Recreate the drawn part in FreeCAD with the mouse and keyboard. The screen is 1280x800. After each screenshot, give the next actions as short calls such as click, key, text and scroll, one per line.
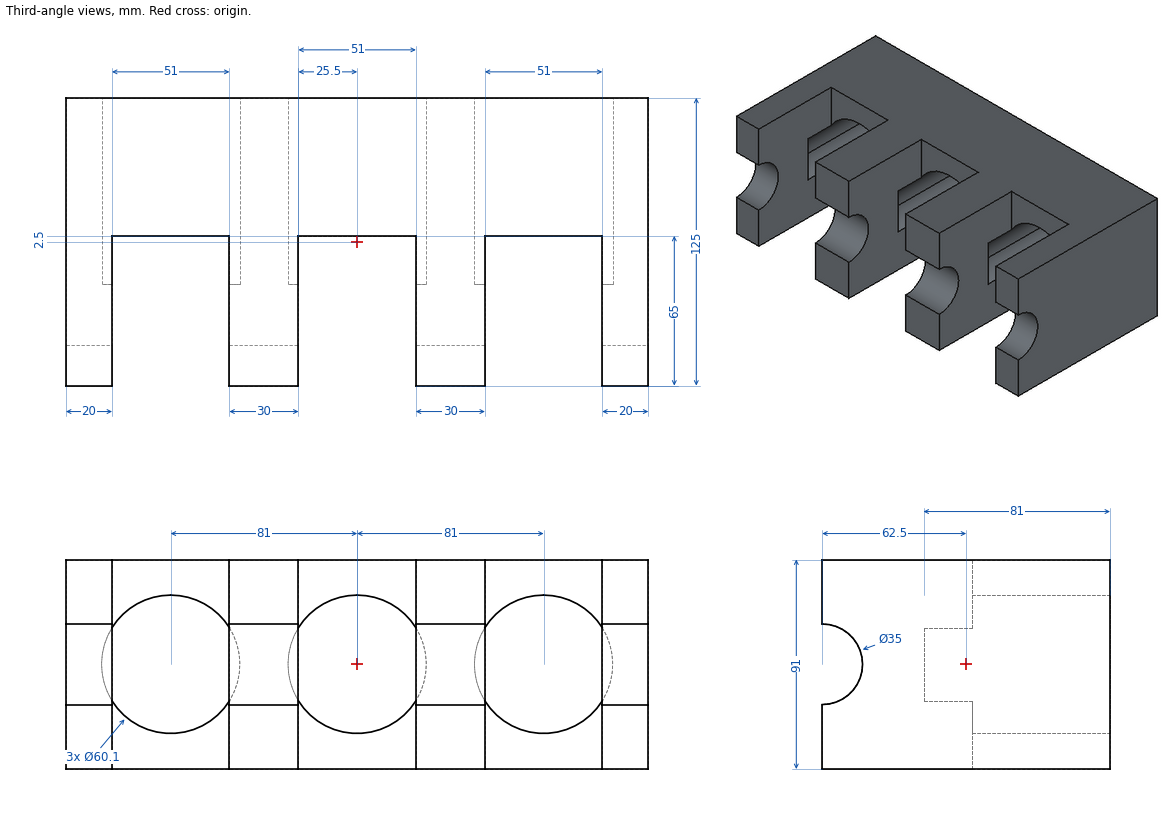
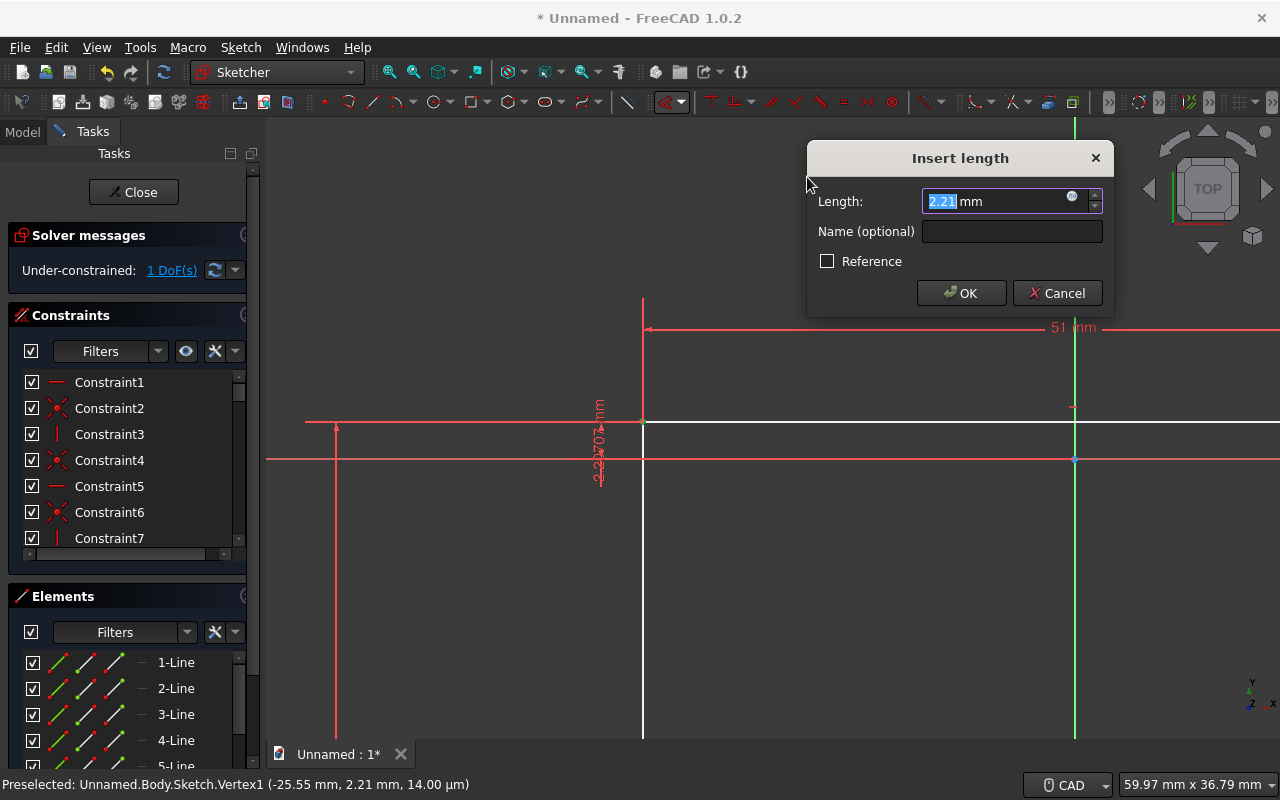
text(2.5)
key(Return)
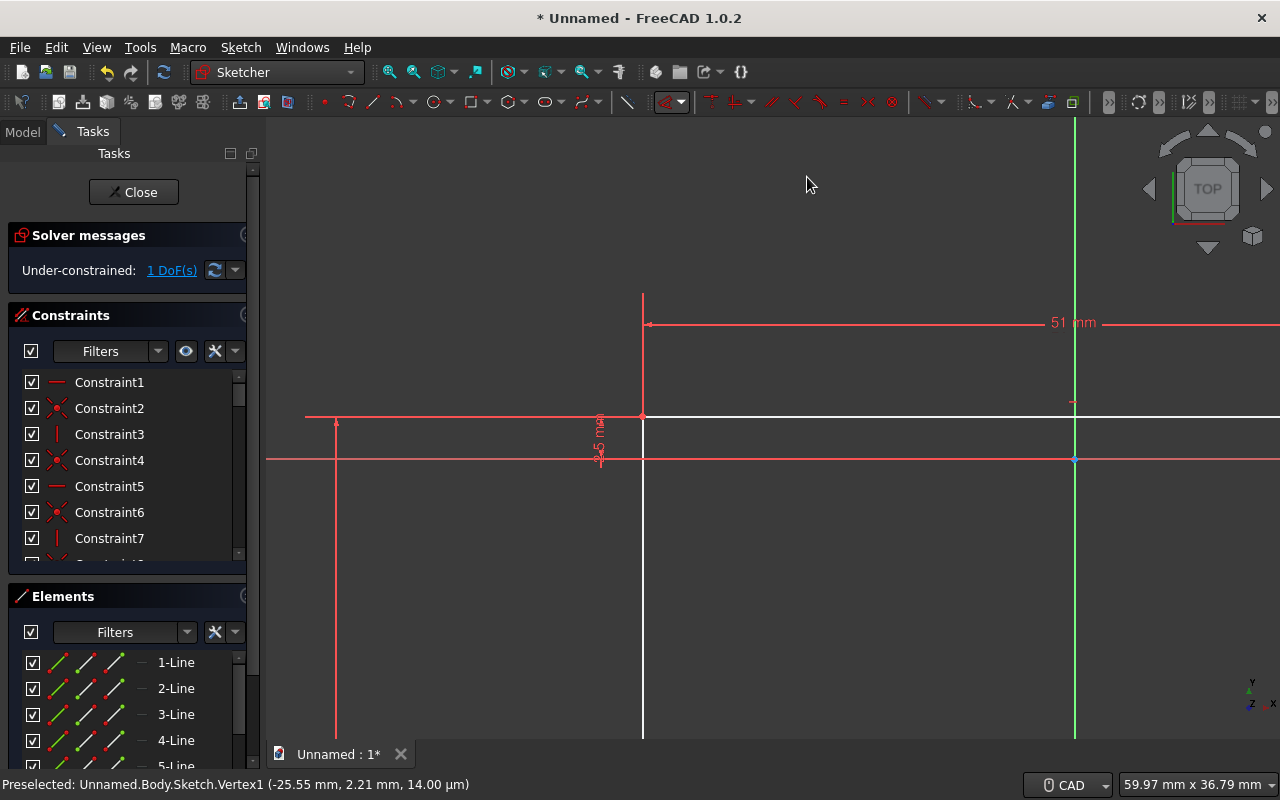
scroll(647, 423, down, 10)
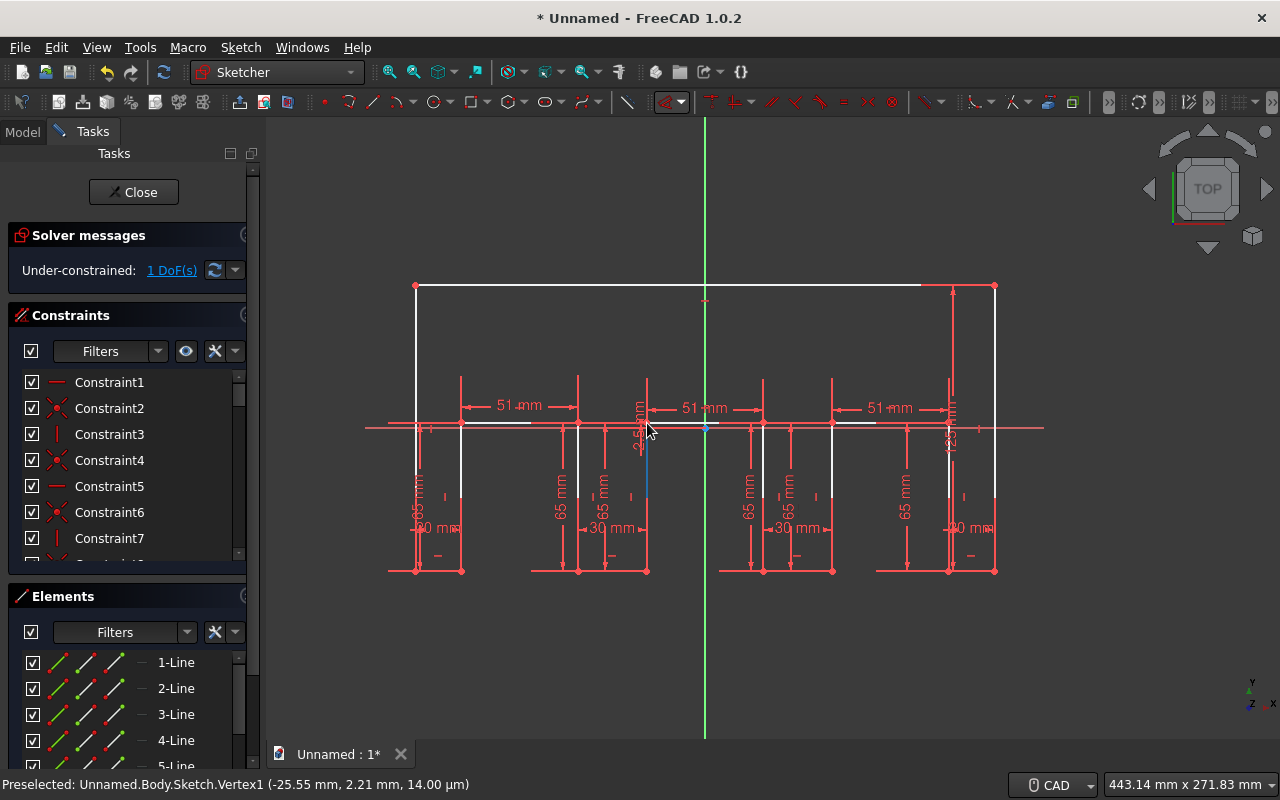
click(647, 423)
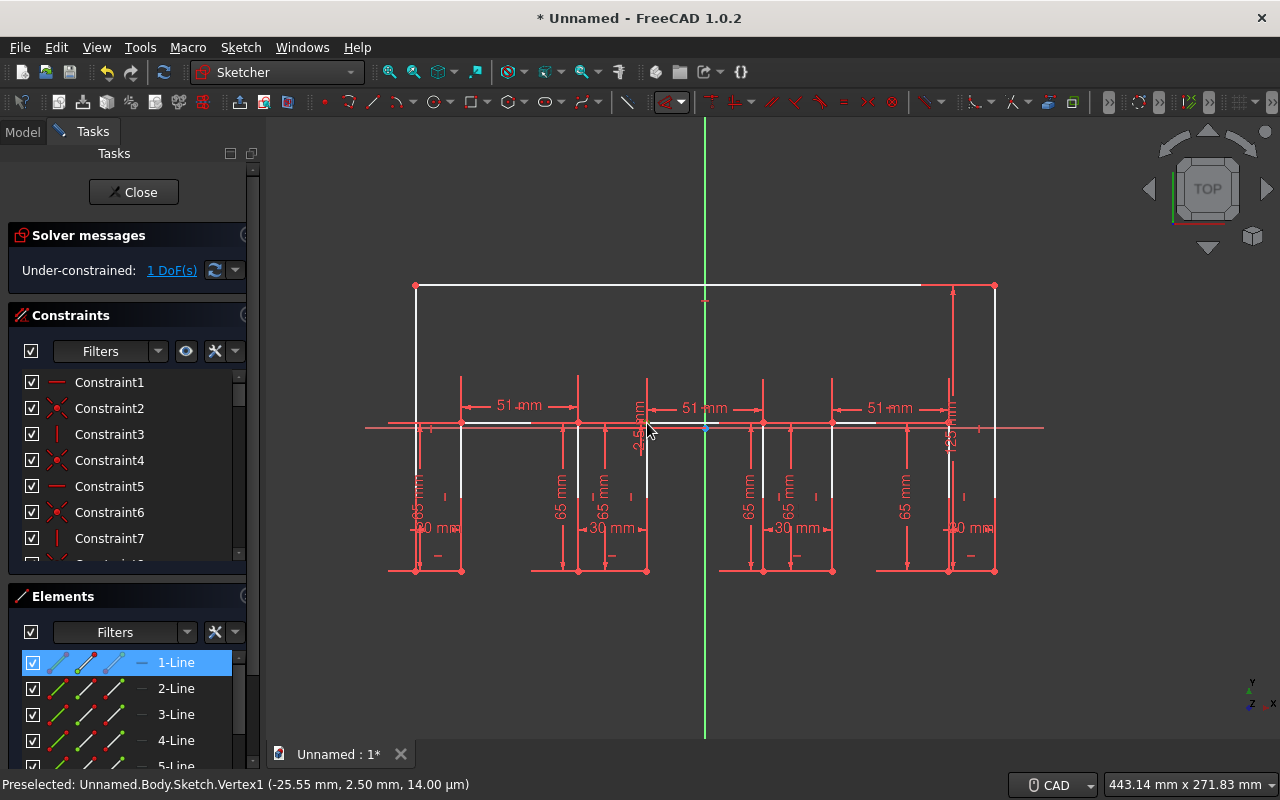
key(l)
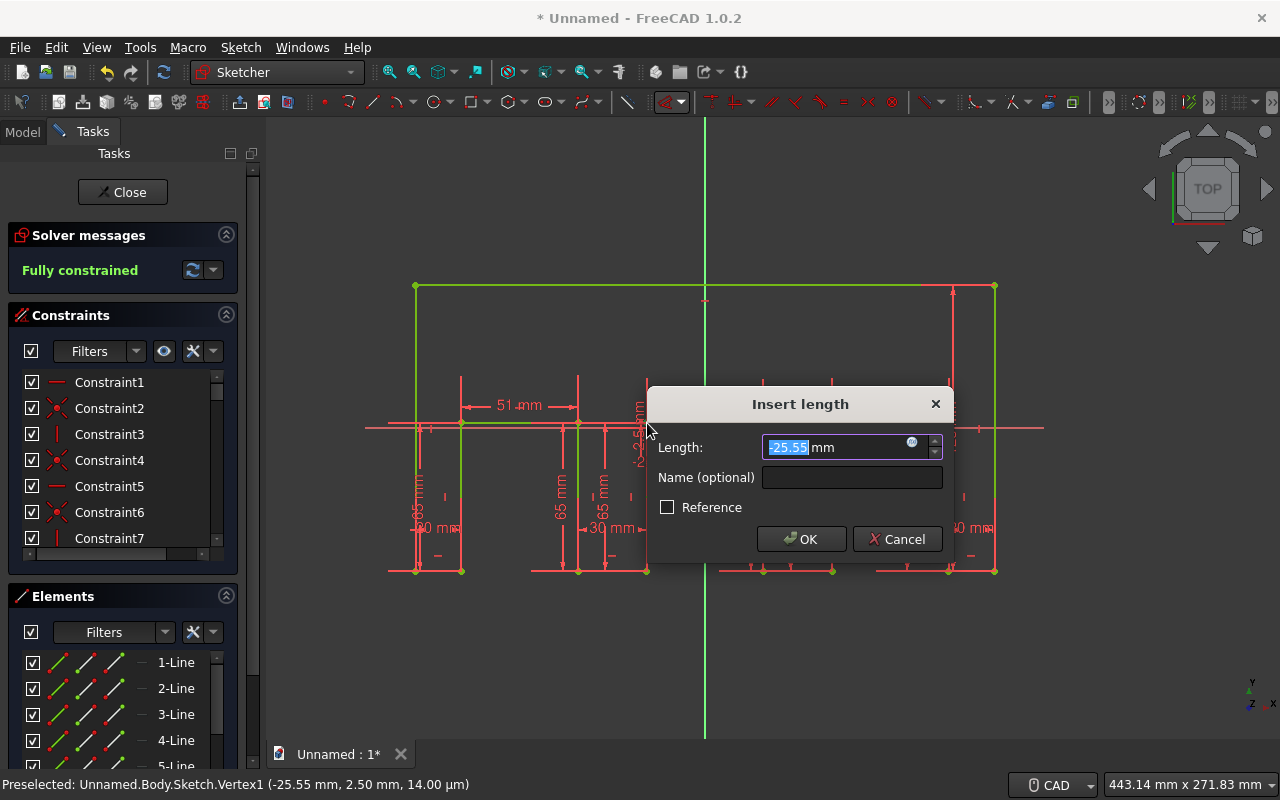
text(-25.5)
key(Return)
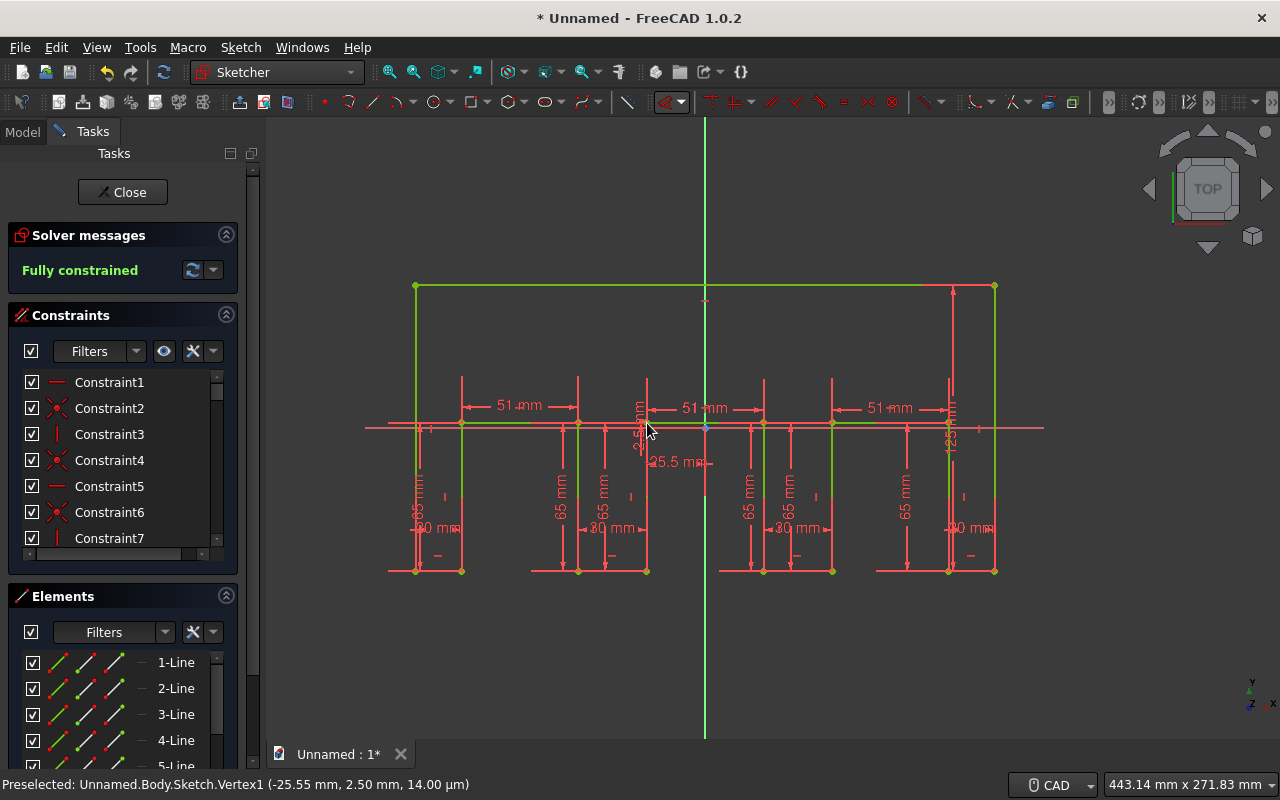
click(123, 192)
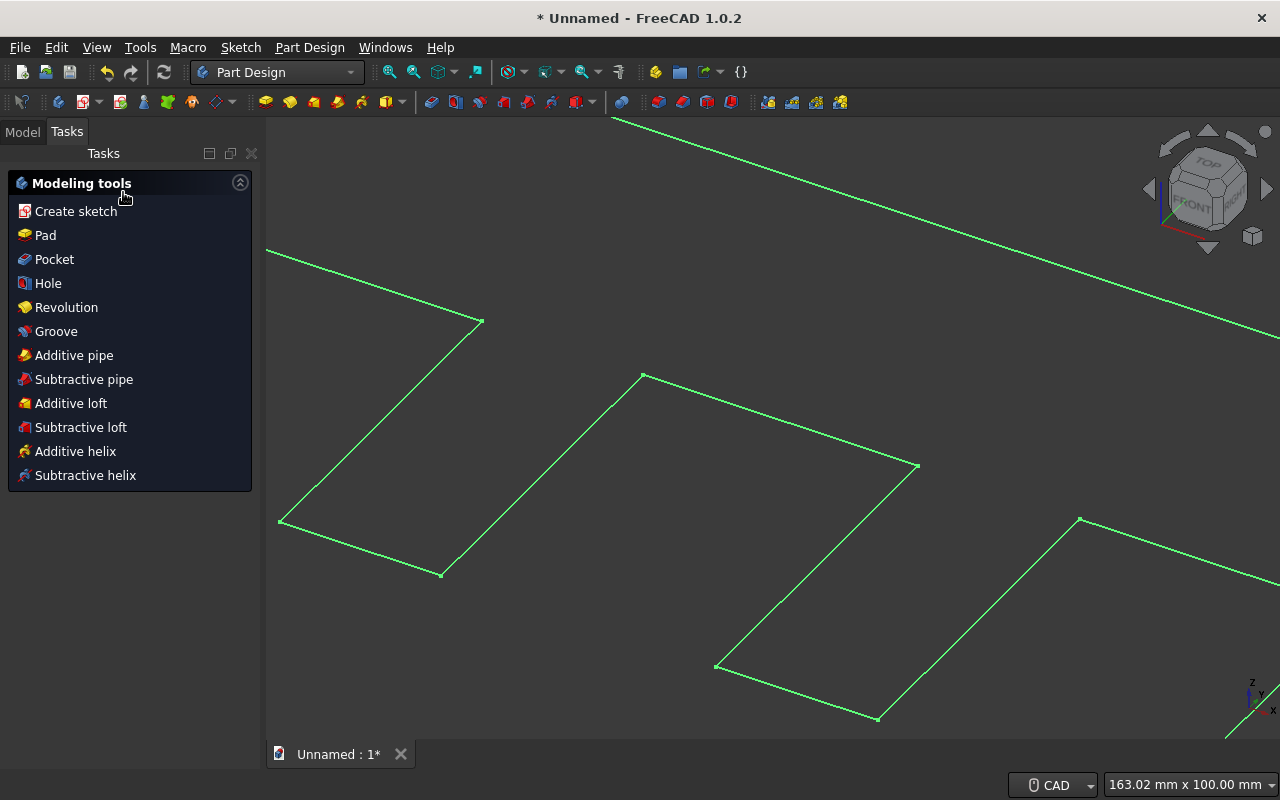
click(266, 102)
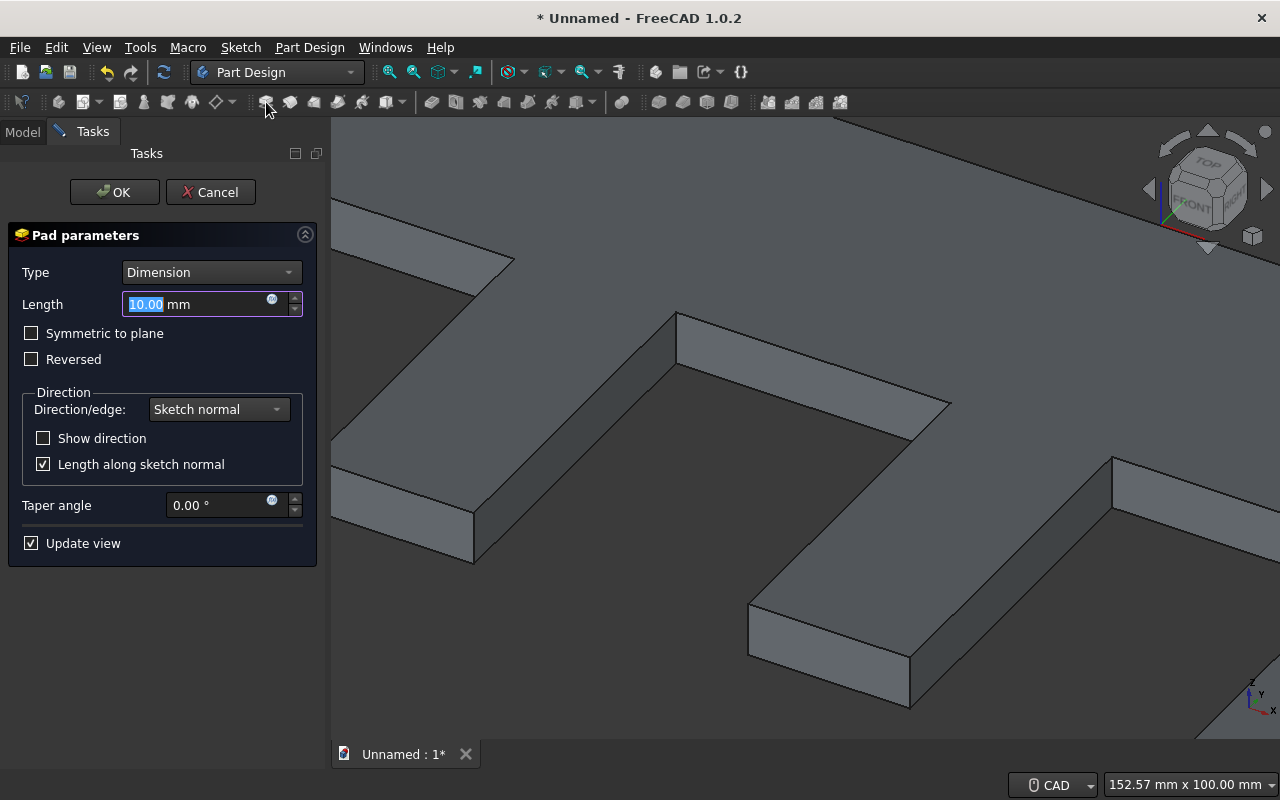
text(91)
key(Tab)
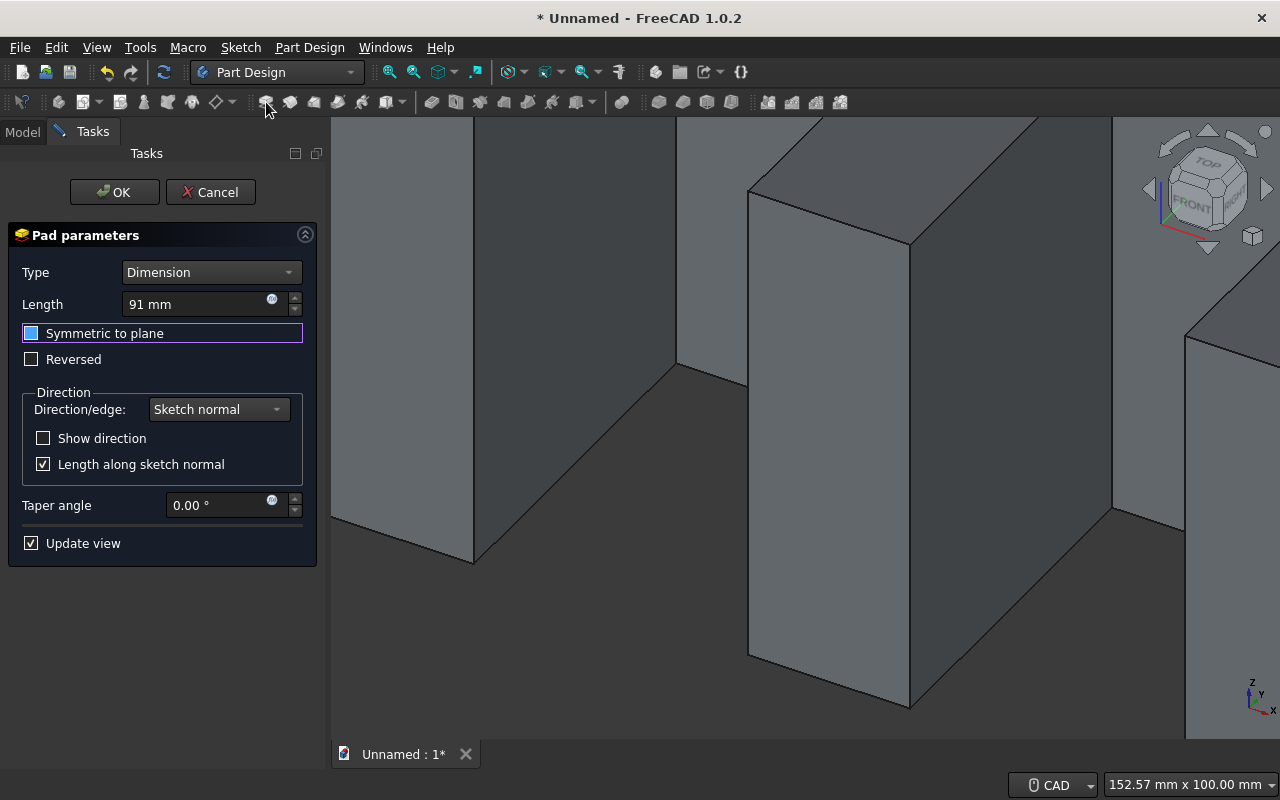
click(30, 333)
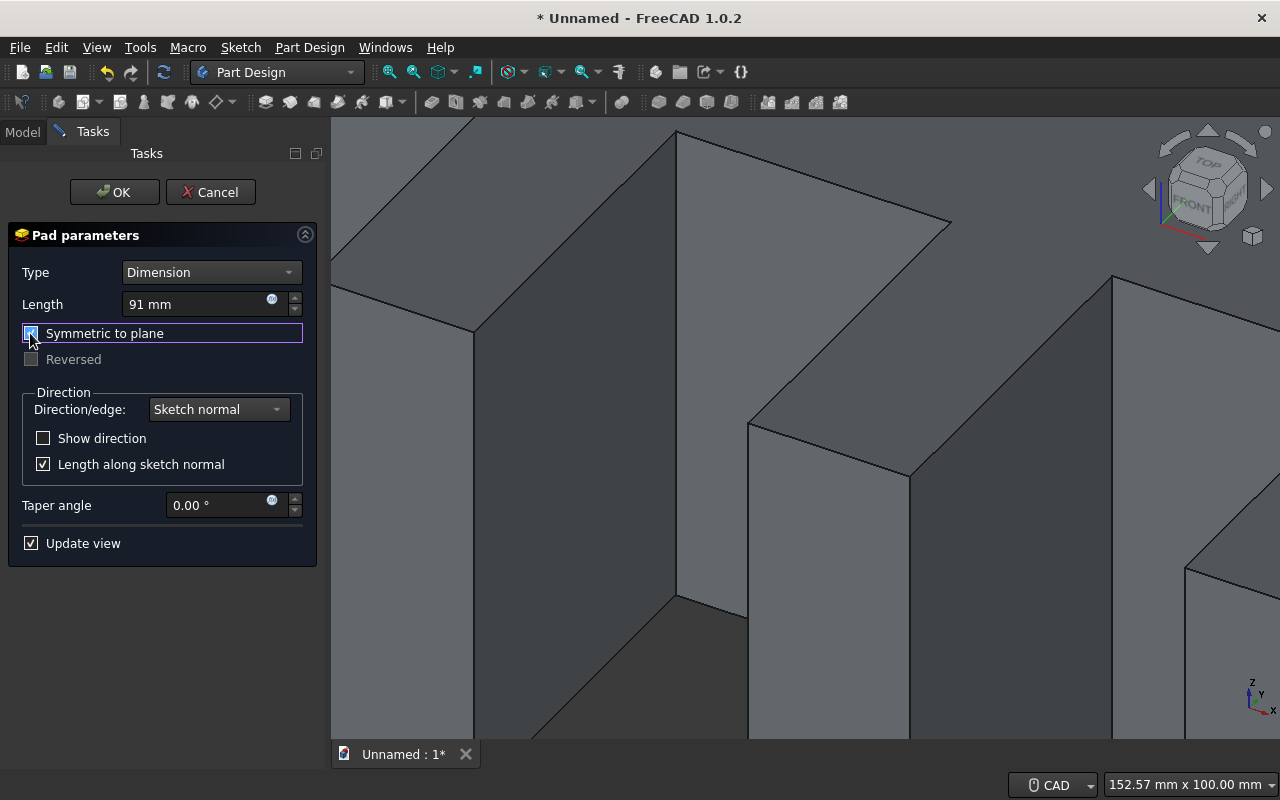
click(115, 192)